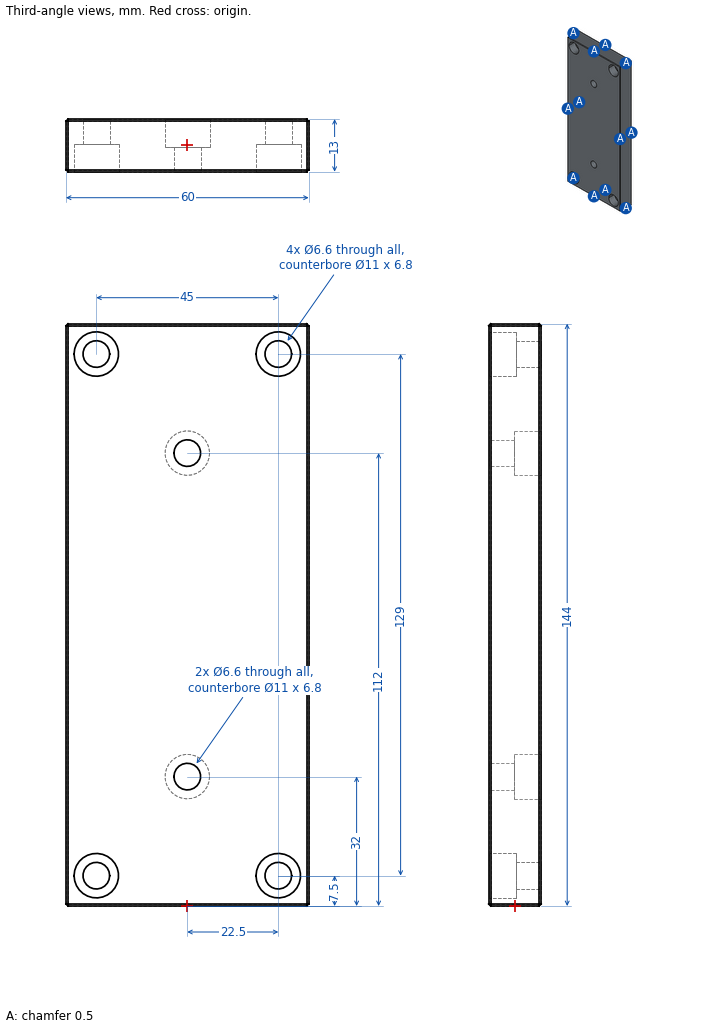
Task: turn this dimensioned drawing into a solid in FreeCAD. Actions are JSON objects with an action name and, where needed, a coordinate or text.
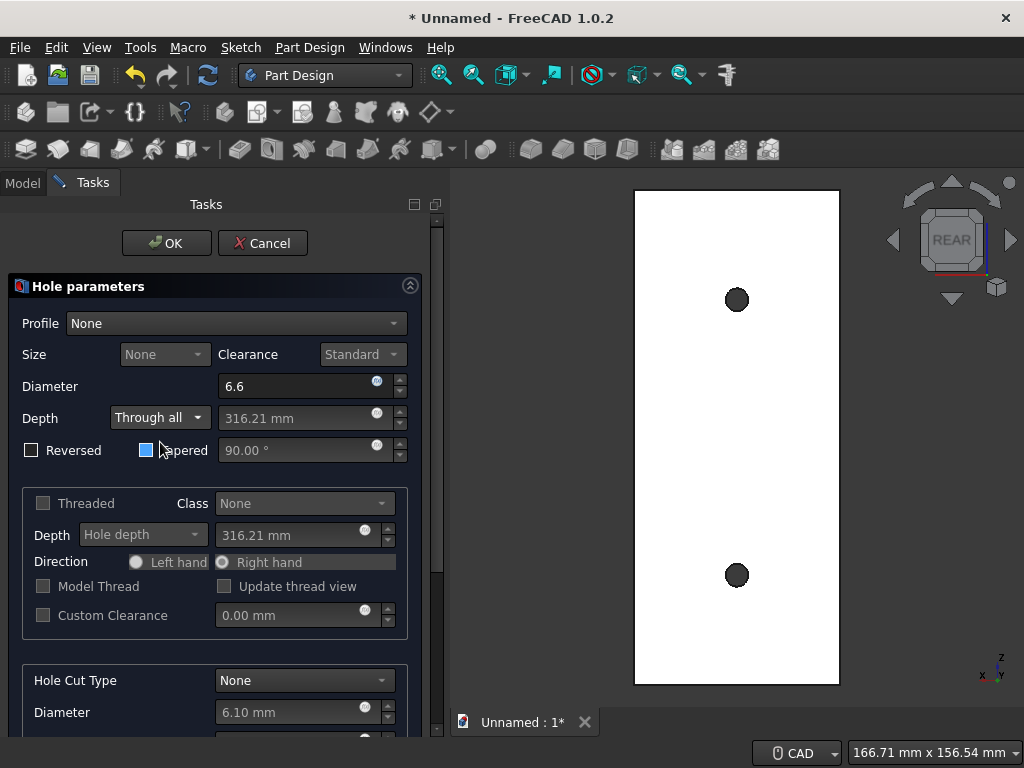
{"action": "left_click", "coordinate": [306, 680]}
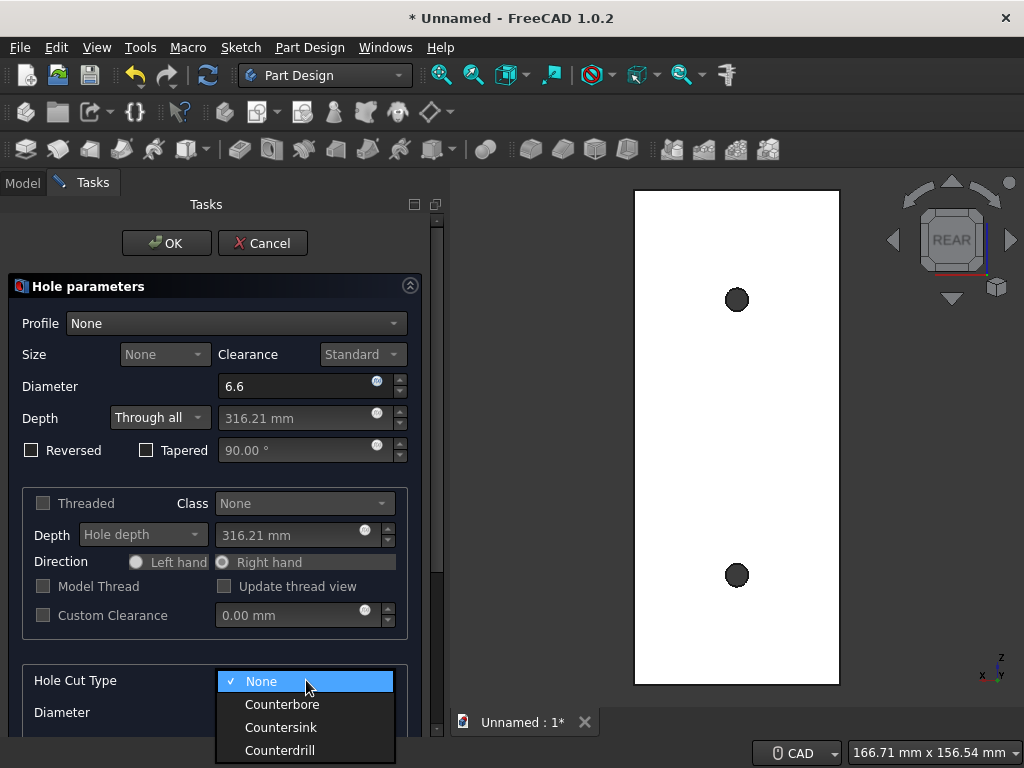
{"action": "left_click", "coordinate": [304, 704]}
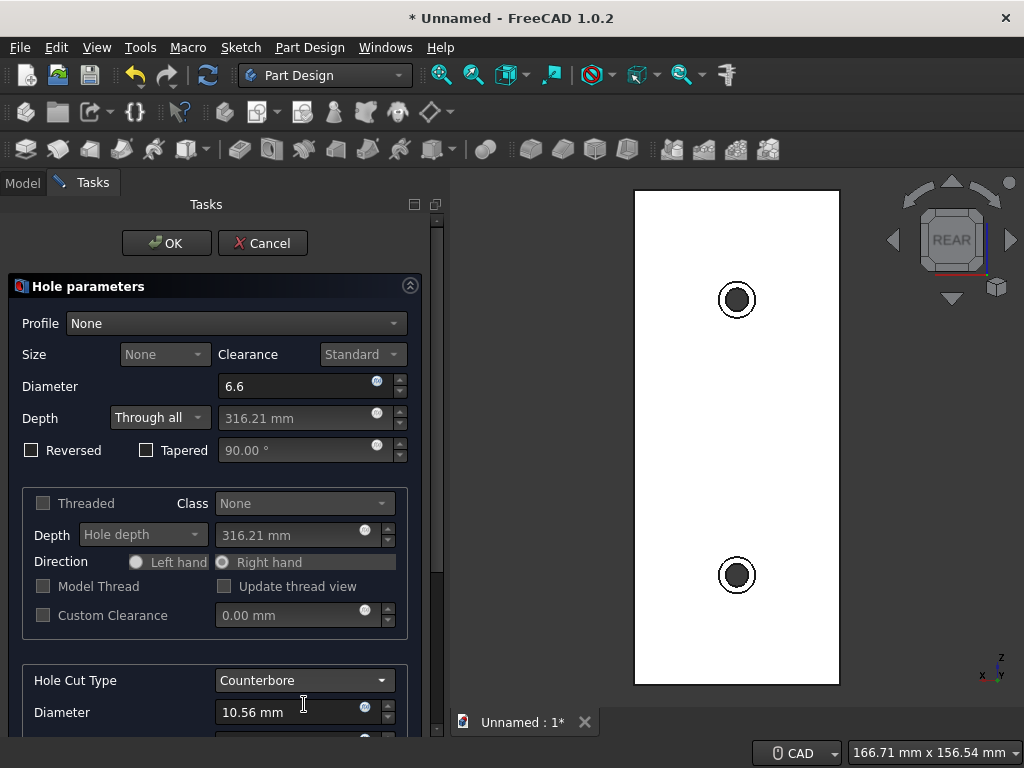
{"action": "triple_click", "coordinate": [298, 712]}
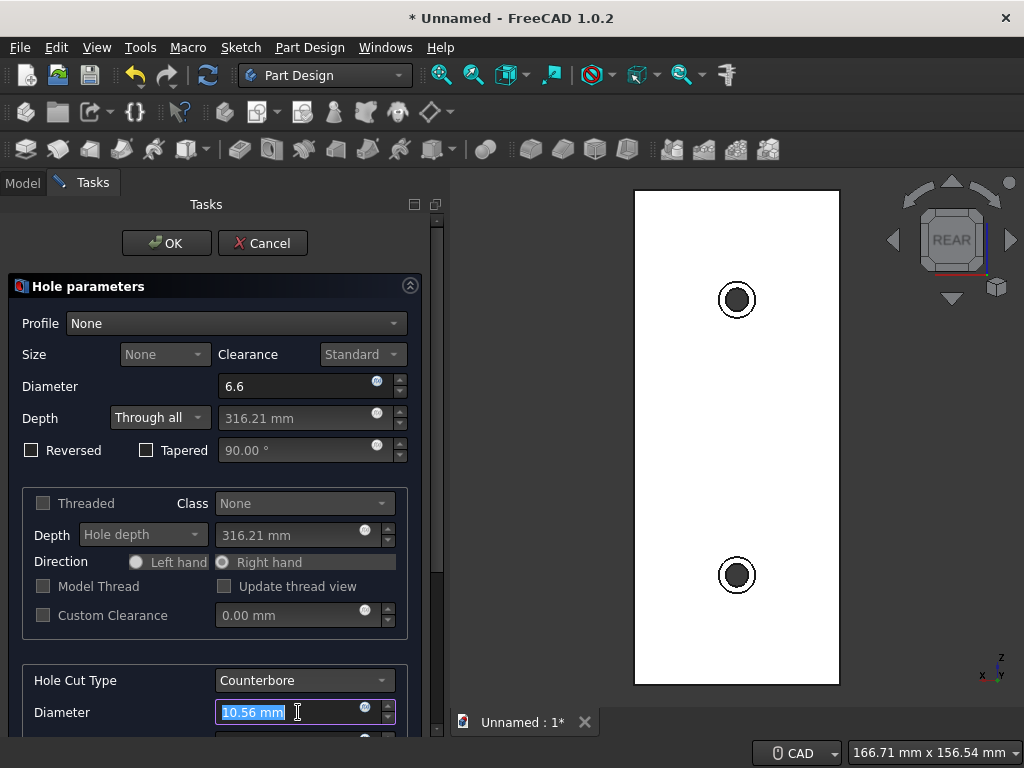
{"action": "type", "text": "11"}
{"action": "key", "text": "Tab"}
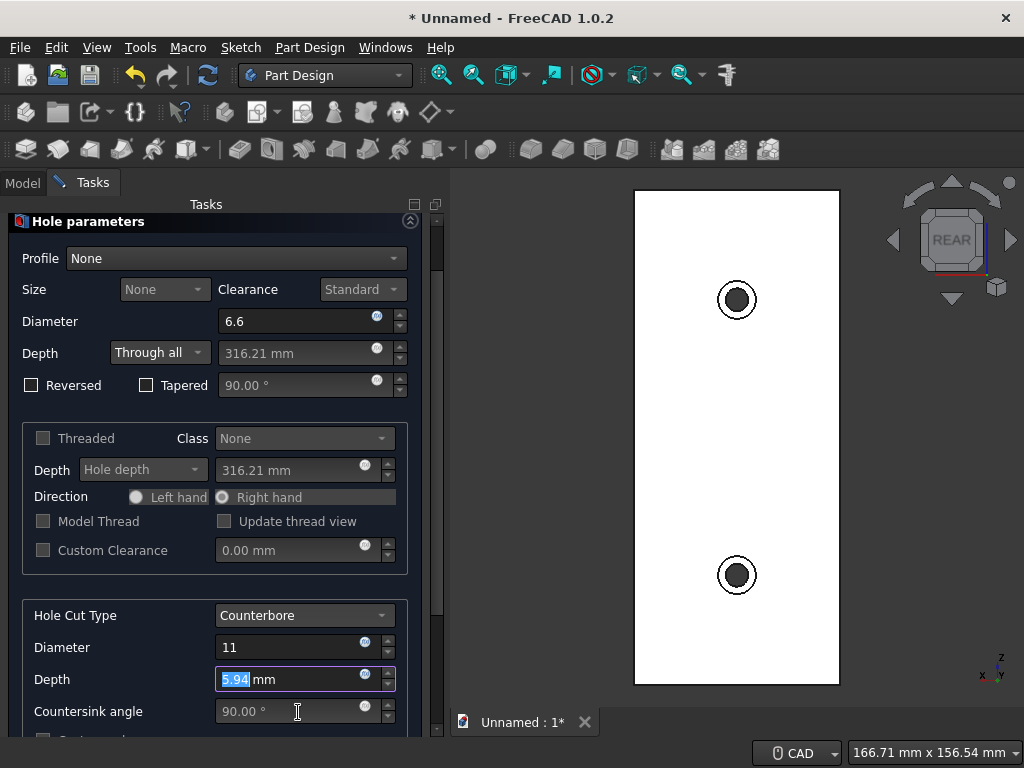
{"action": "type", "text": "6.8"}
{"action": "key", "text": "Tab"}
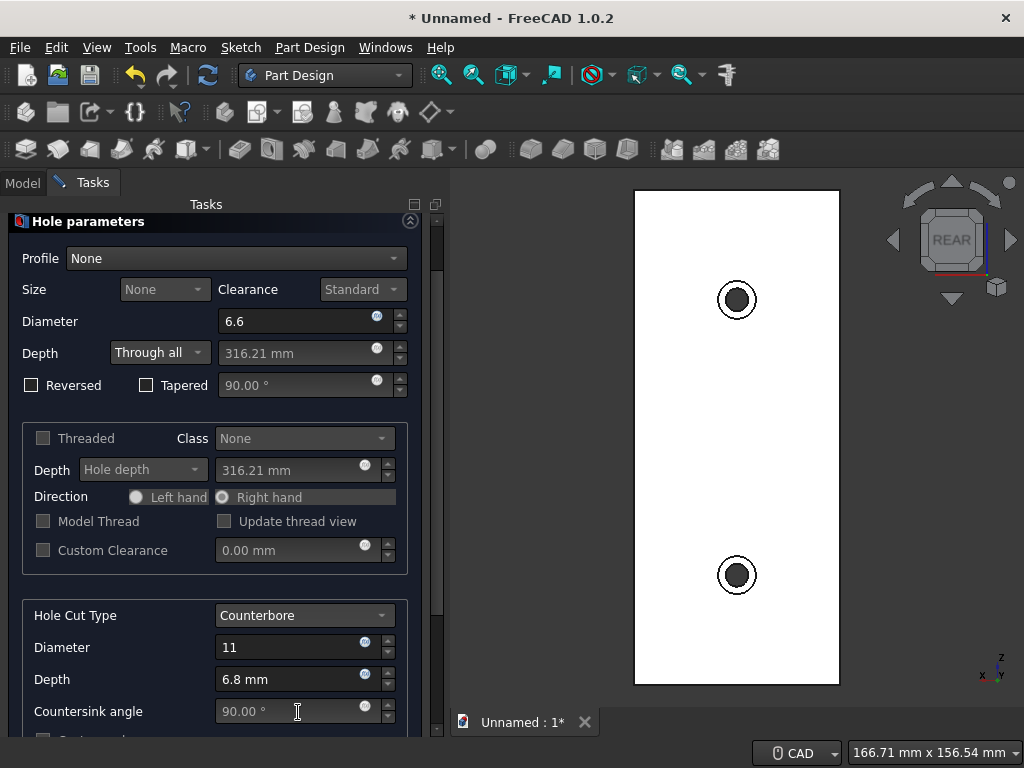
{"action": "scroll", "coordinate": [437, 475], "scroll_direction": "up", "scroll_amount": 2}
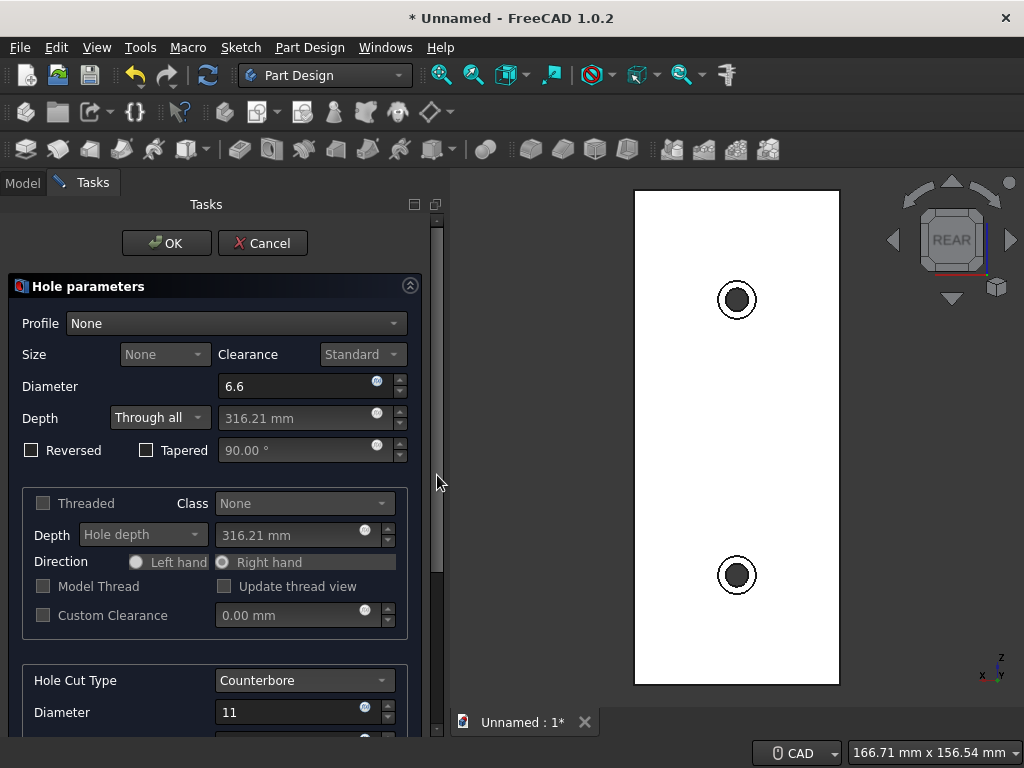
{"action": "left_click", "coordinate": [167, 243]}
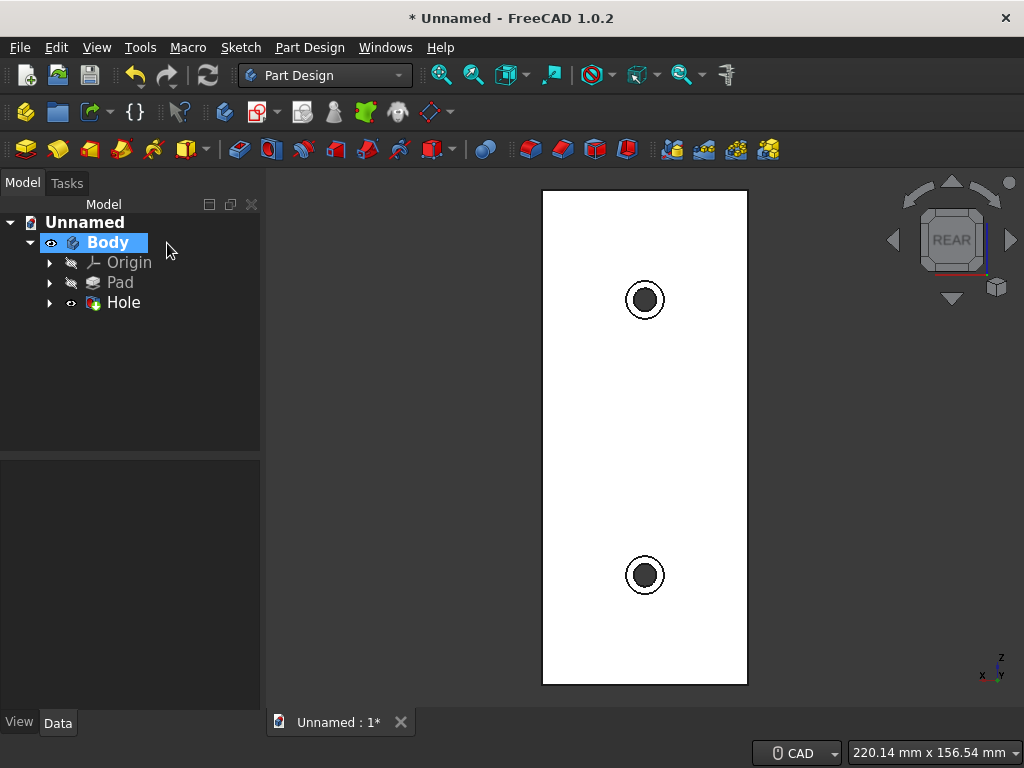
{"action": "key", "text": "0"}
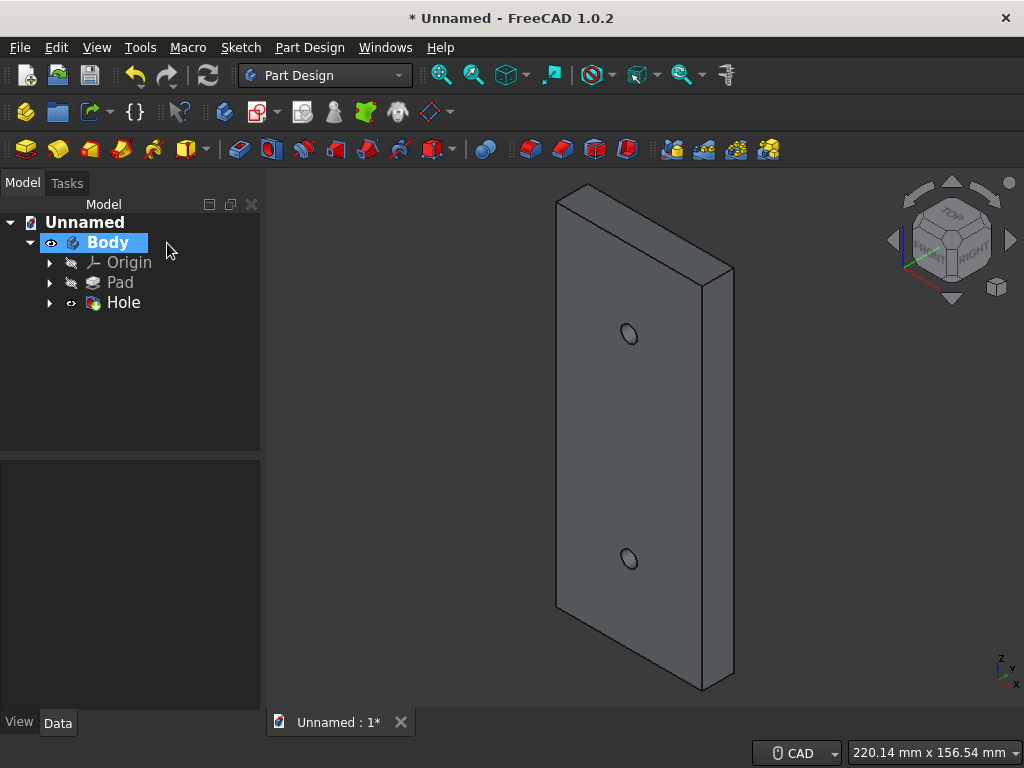
{"action": "left_click", "coordinate": [718, 305]}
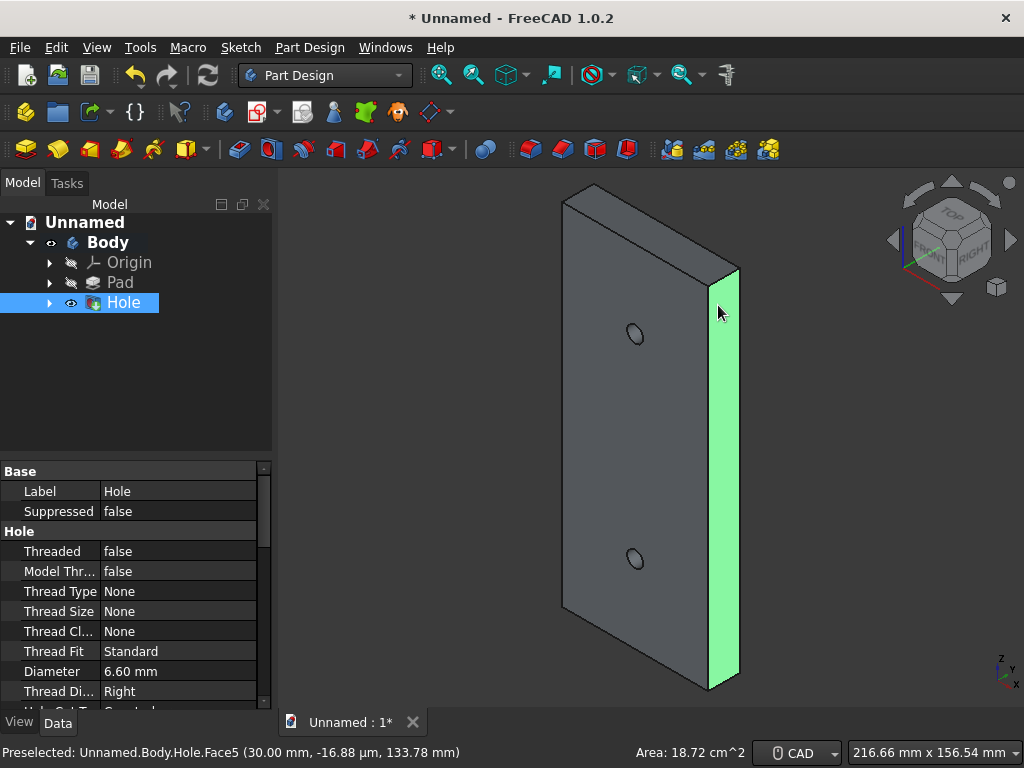
{"action": "left_click", "coordinate": [635, 243], "text": "ctrl"}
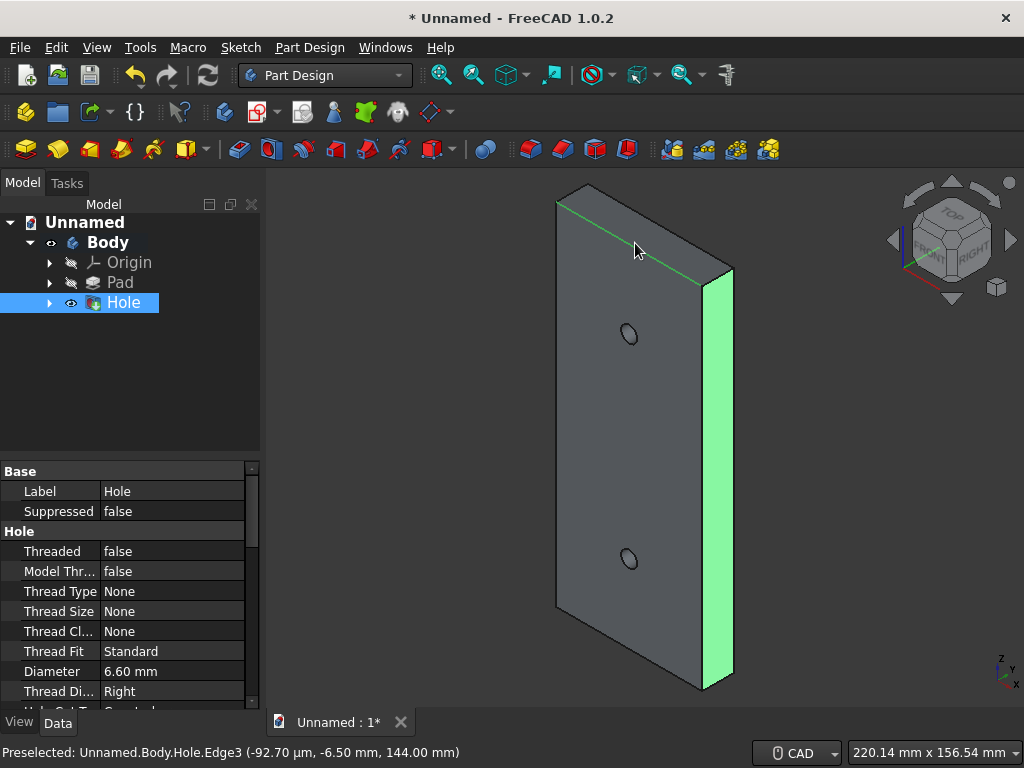
{"action": "key", "text": "2"}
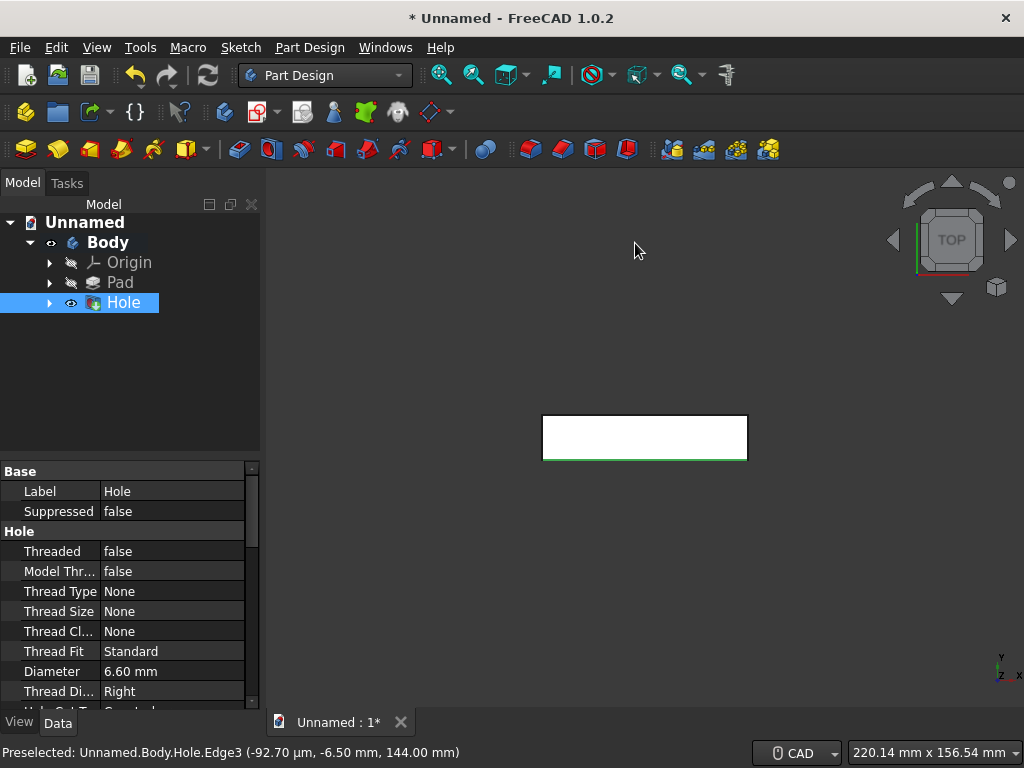
{"action": "key", "text": "v f"}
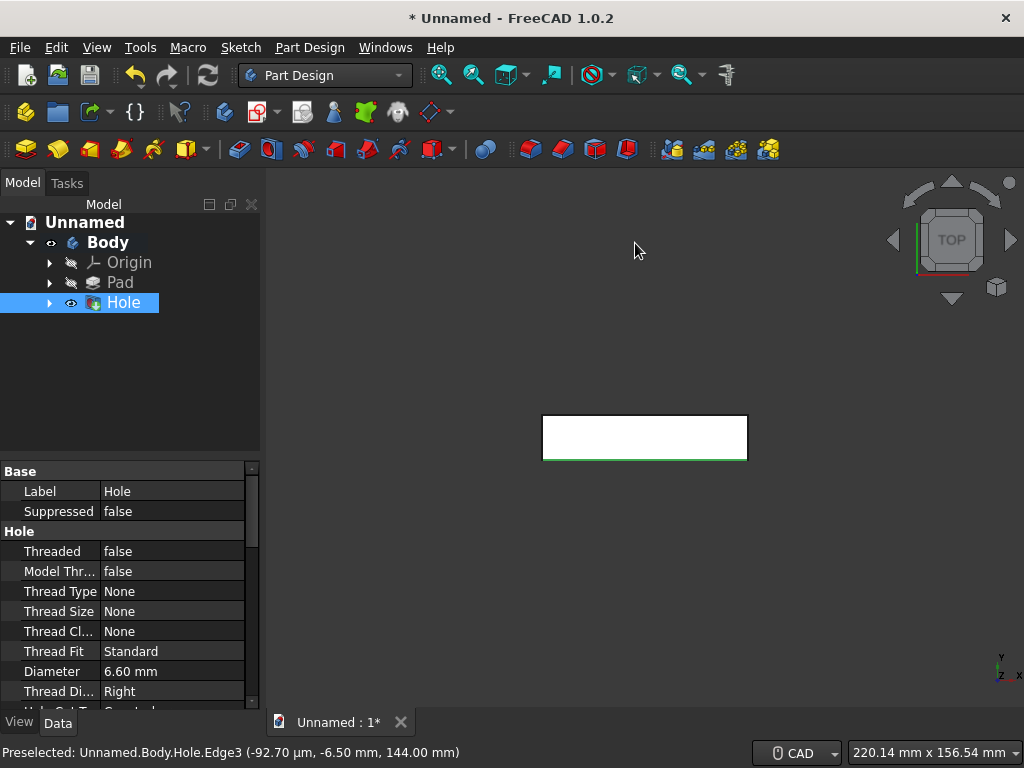
{"action": "left_click", "coordinate": [645, 414], "text": "ctrl"}